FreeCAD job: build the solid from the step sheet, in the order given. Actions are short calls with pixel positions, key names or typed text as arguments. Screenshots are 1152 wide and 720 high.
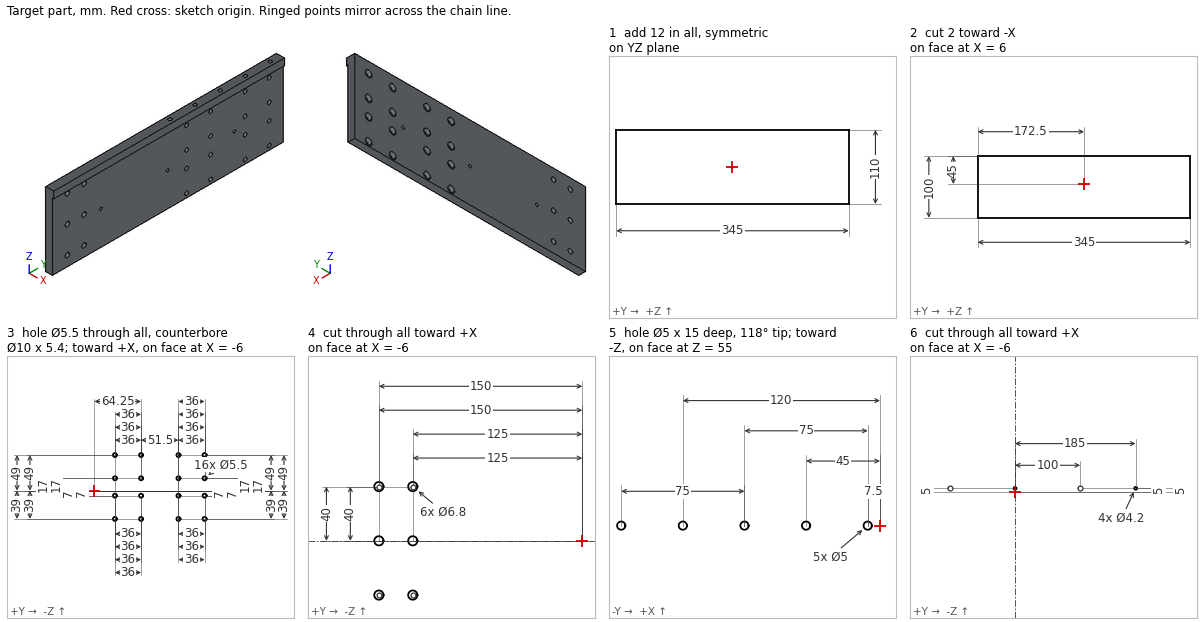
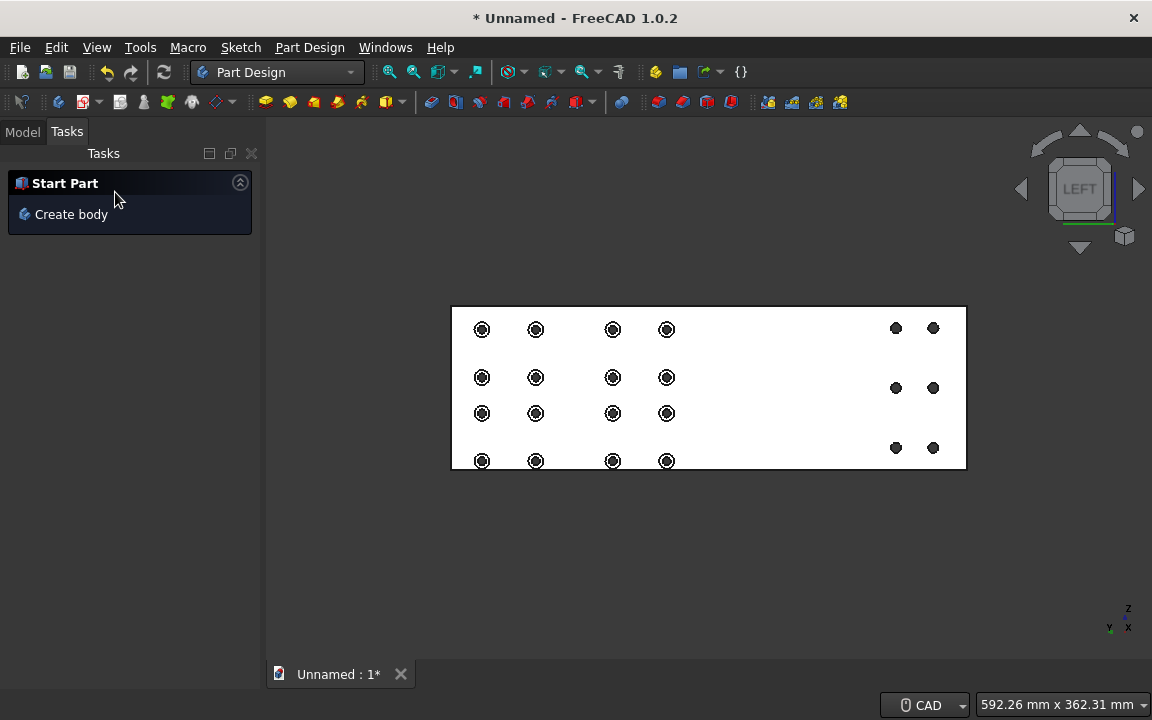
key(0)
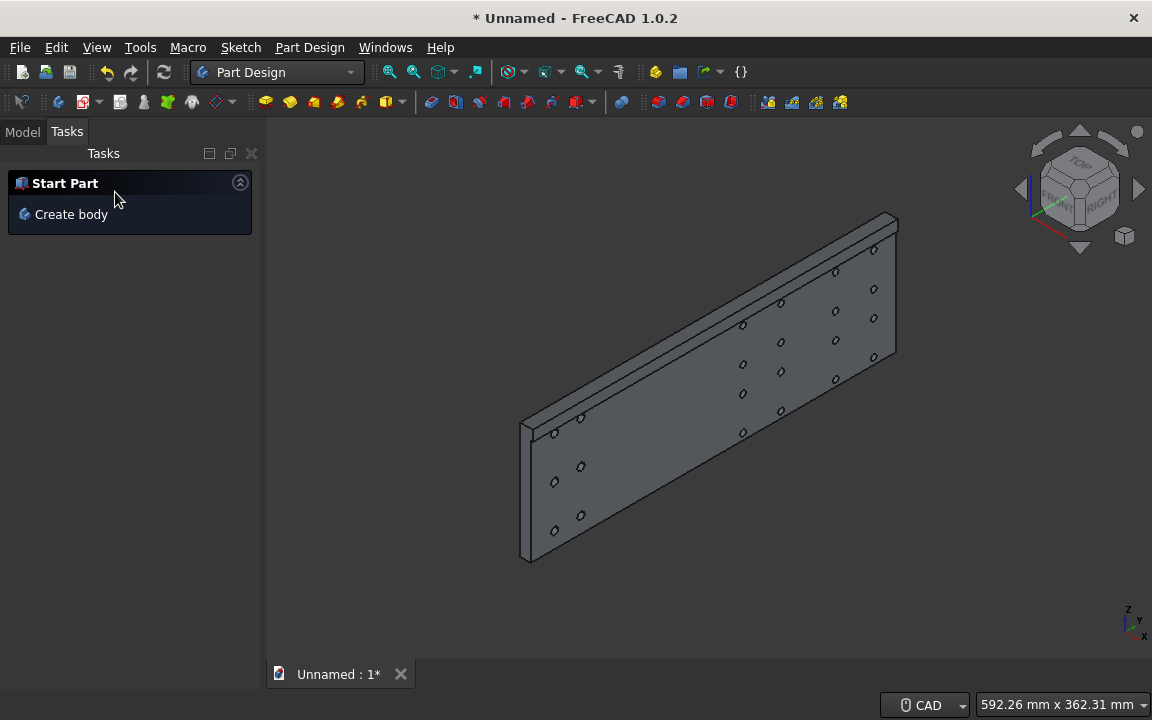
key(2)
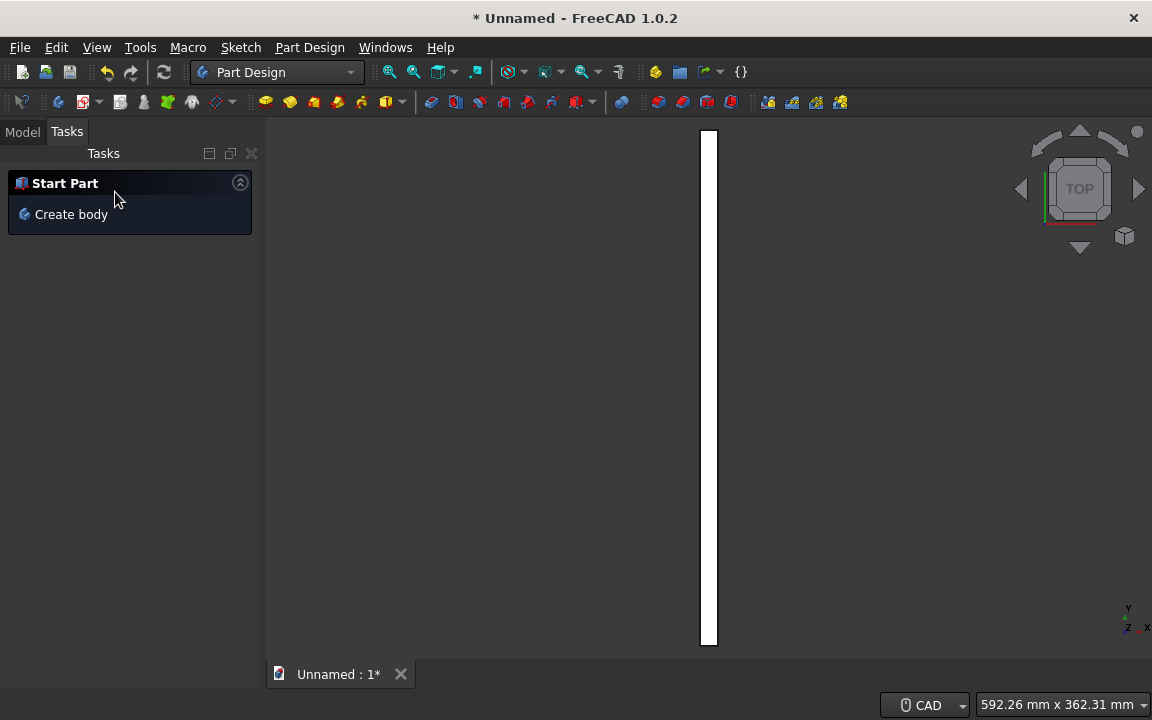
click(709, 166)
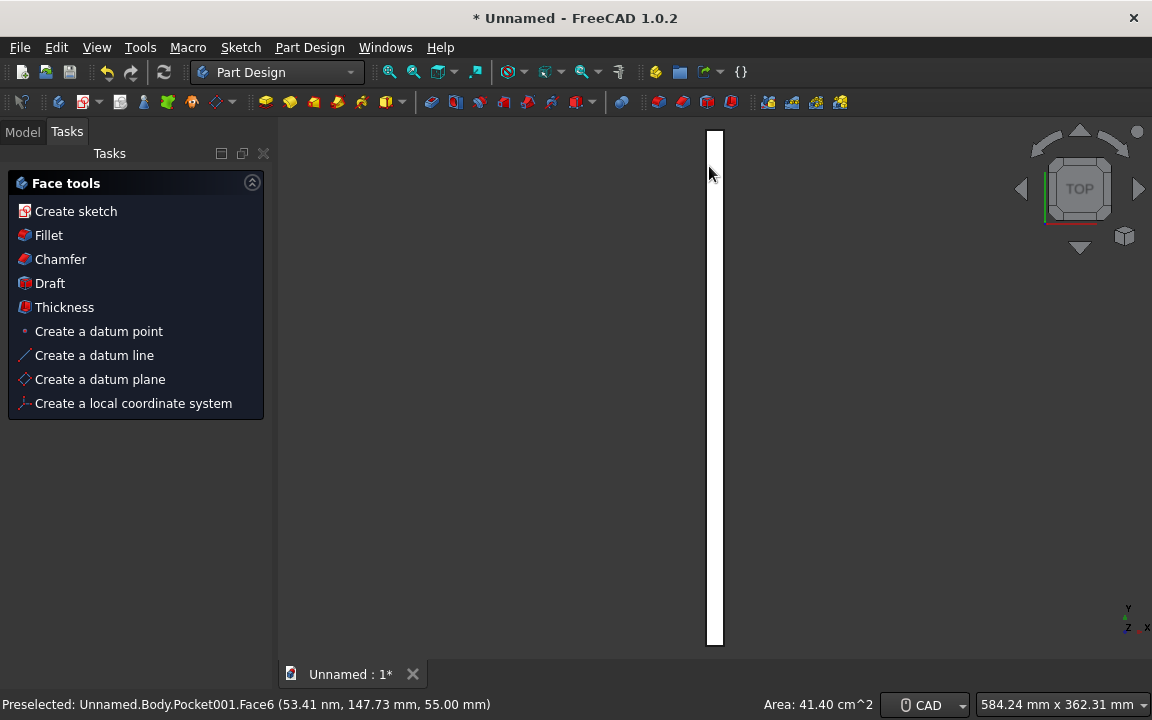
click(84, 102)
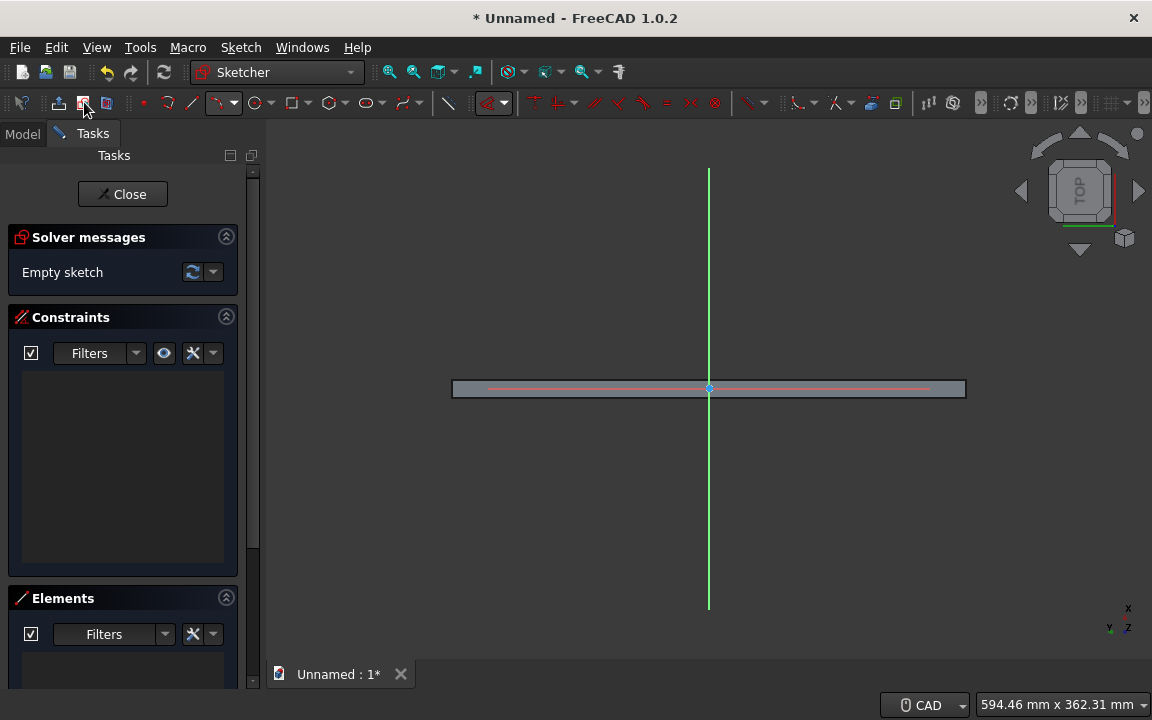
scroll(548, 389, up, 4)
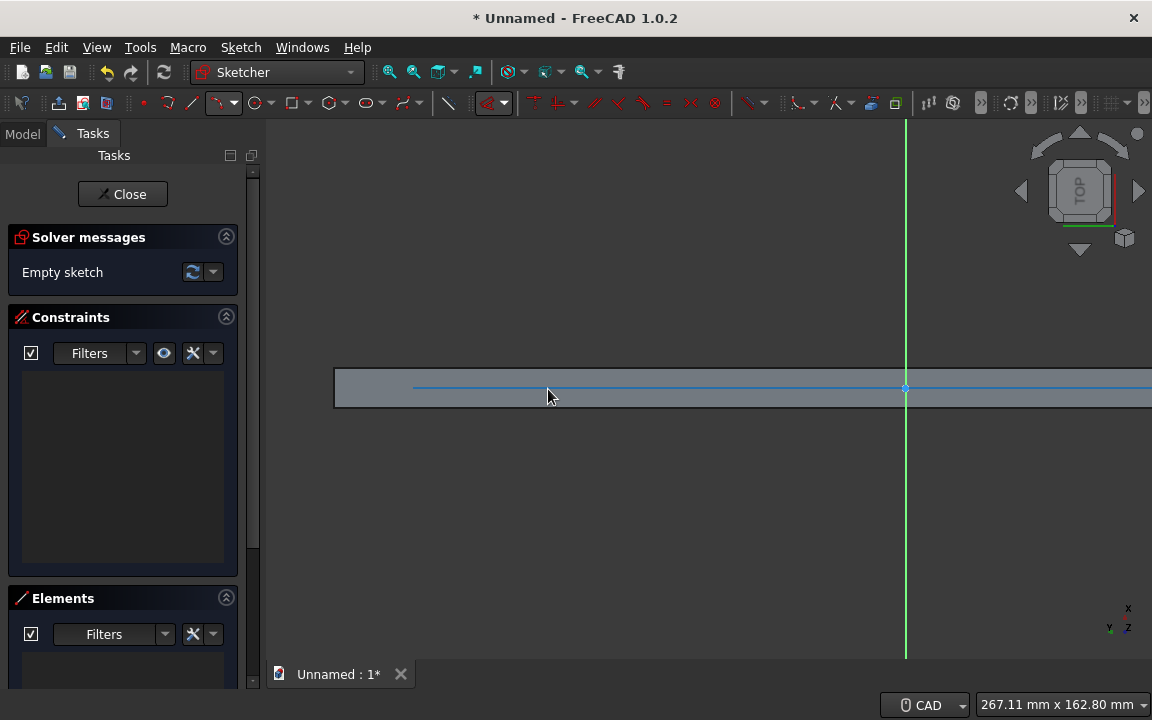
click(256, 104)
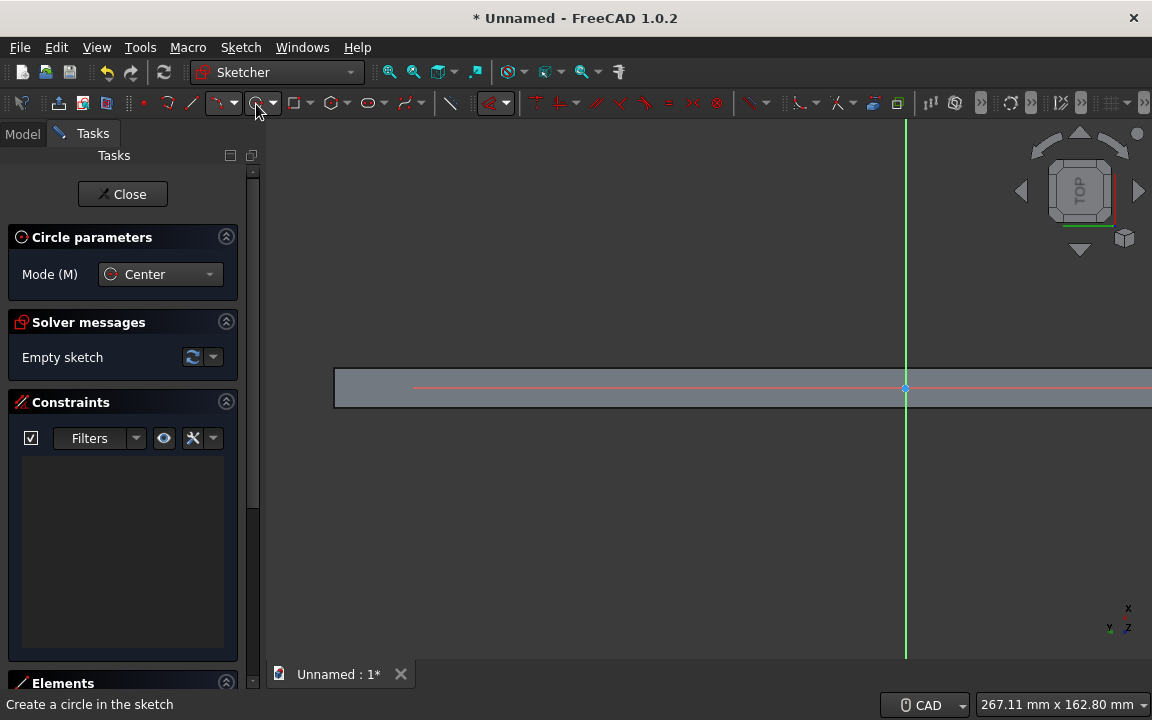
scroll(881, 388, up, 6)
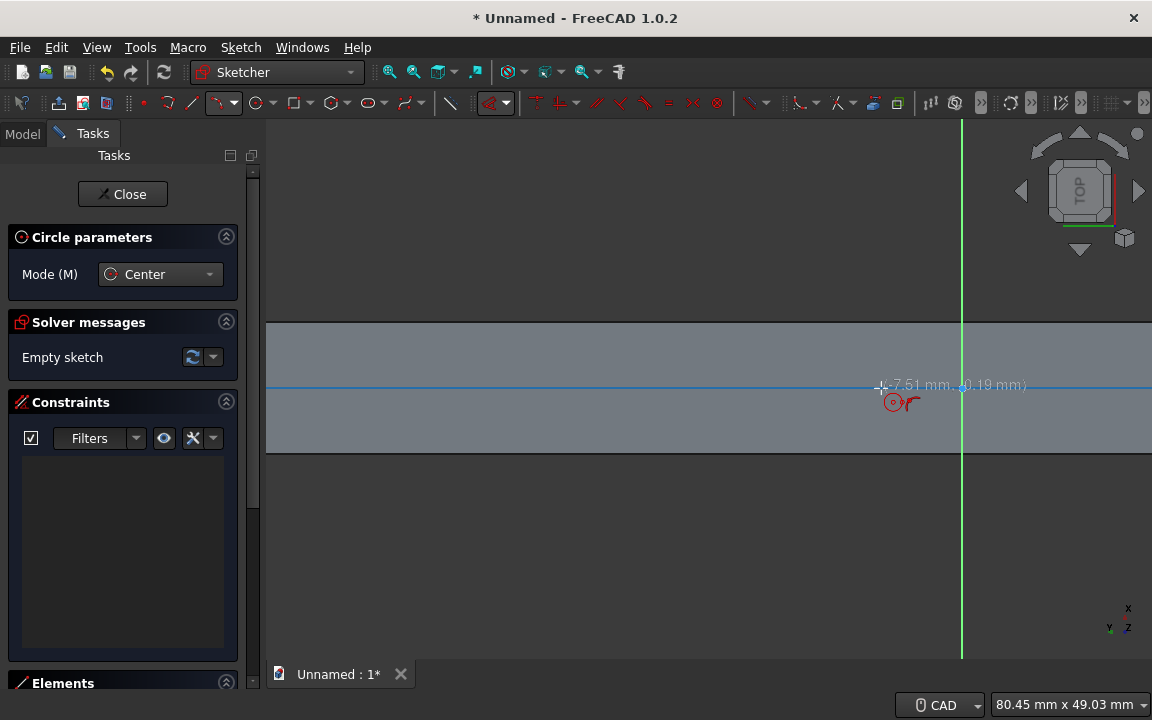
click(880, 388)
click(899, 369)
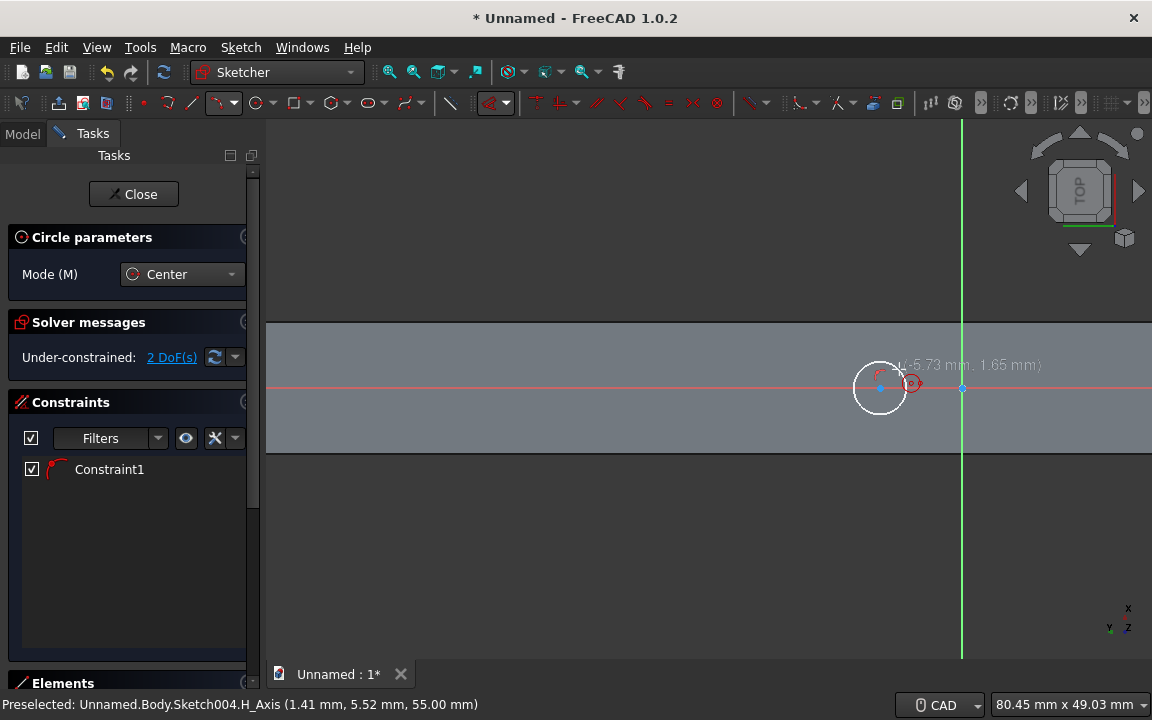
click(467, 388)
click(486, 369)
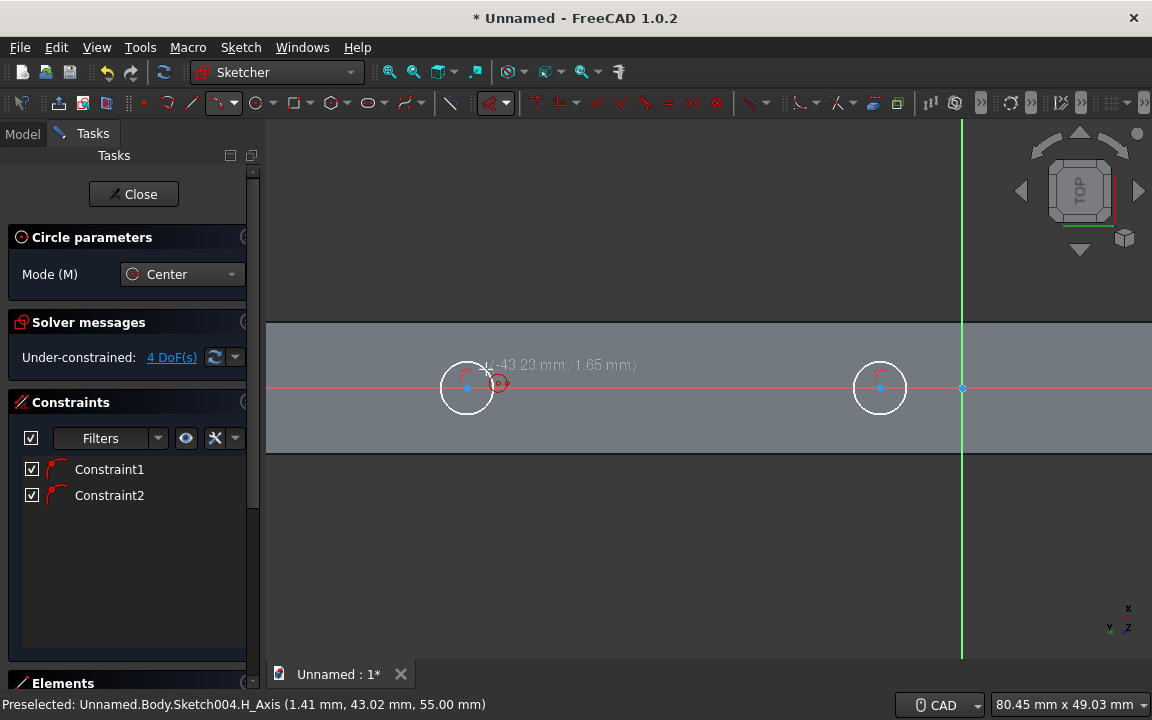
scroll(882, 389, down, 6)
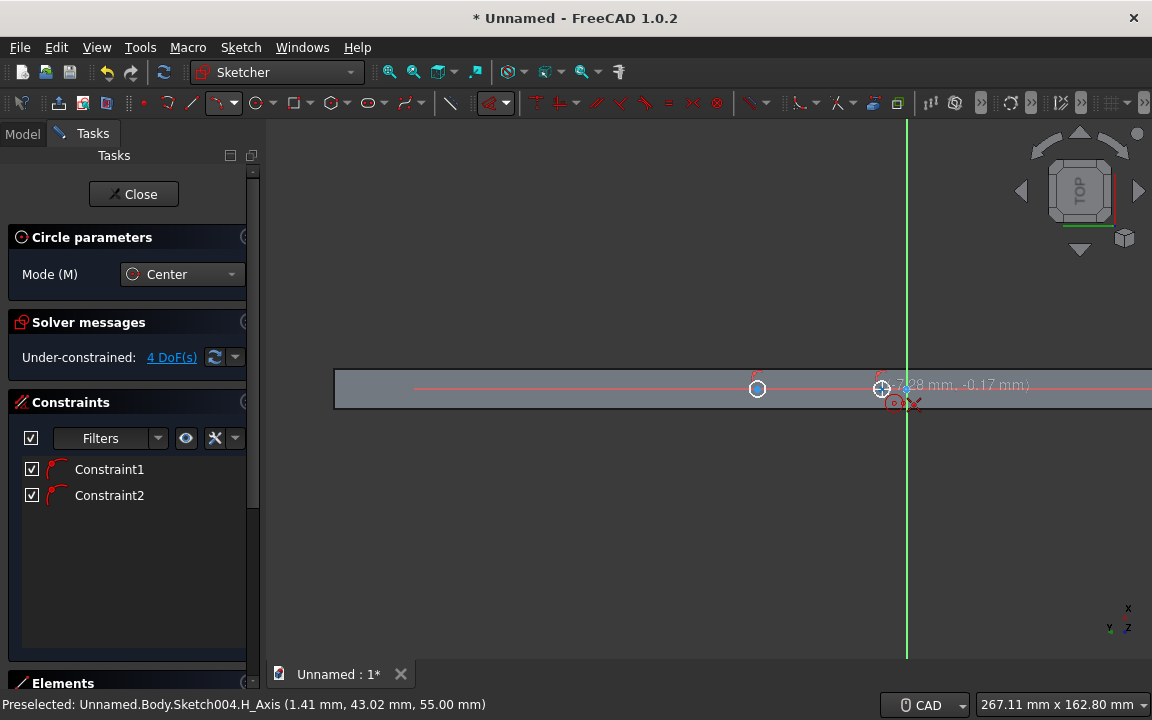
scroll(633, 389, up, 6)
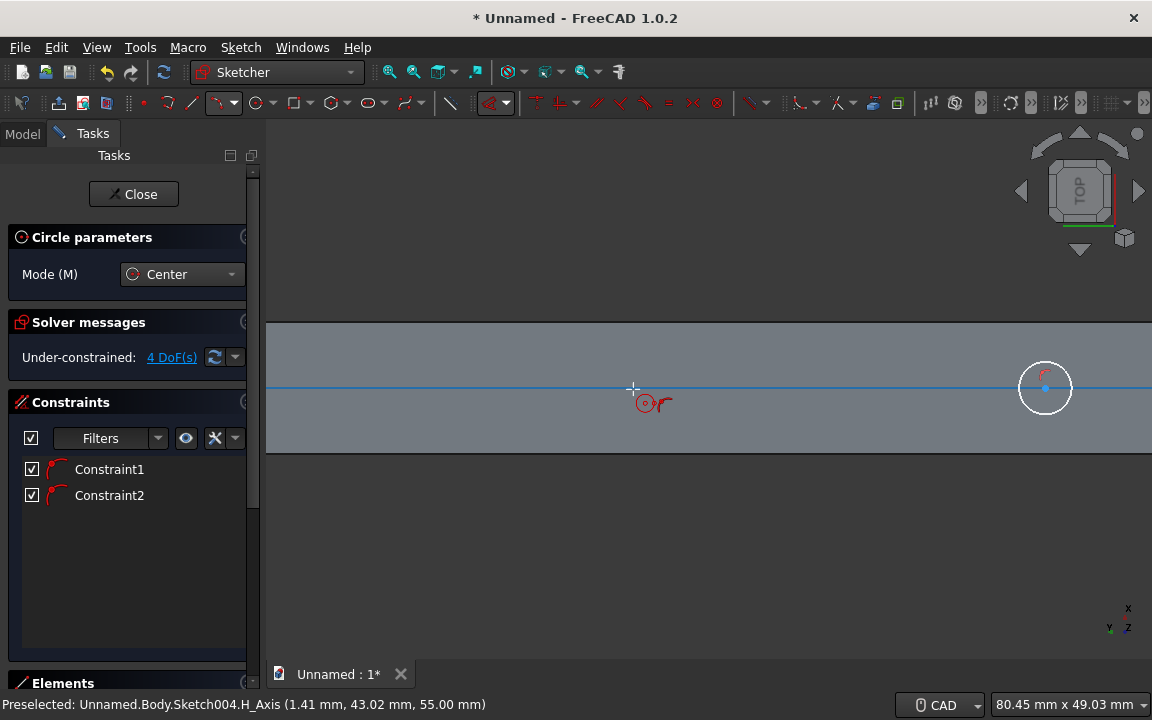
click(632, 388)
click(651, 369)